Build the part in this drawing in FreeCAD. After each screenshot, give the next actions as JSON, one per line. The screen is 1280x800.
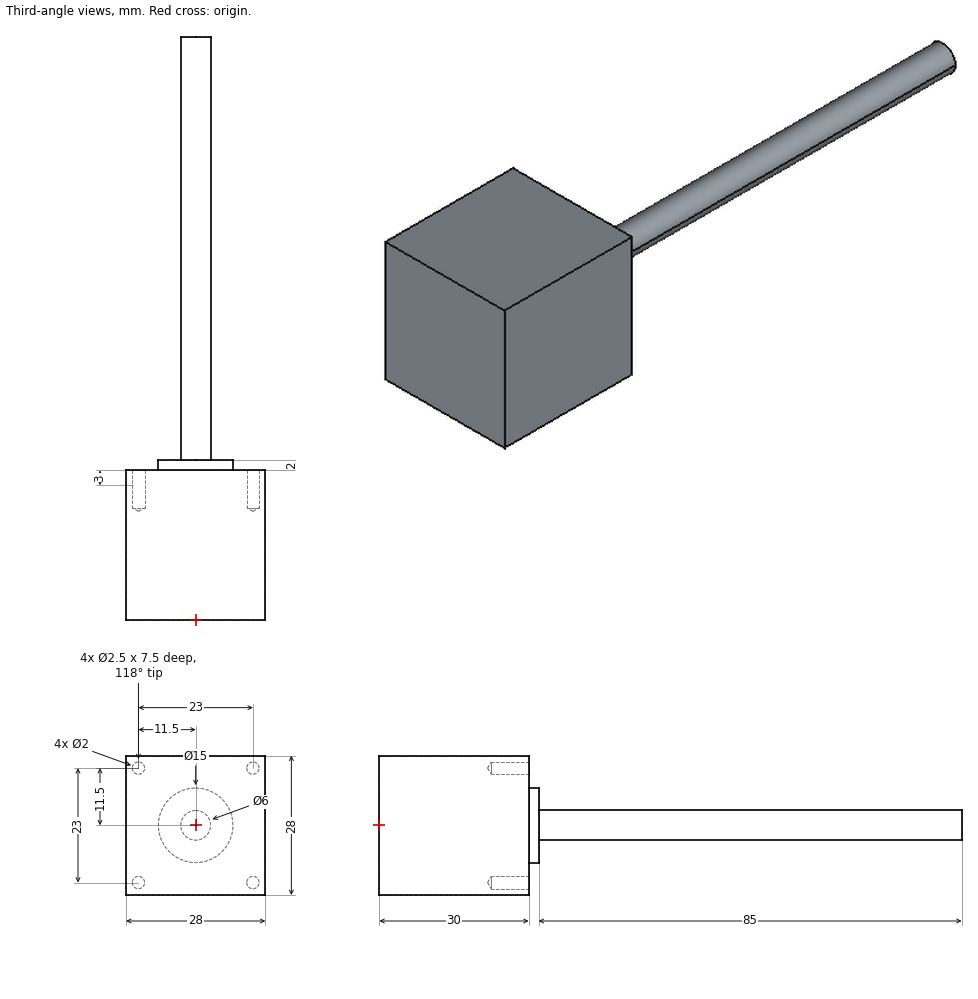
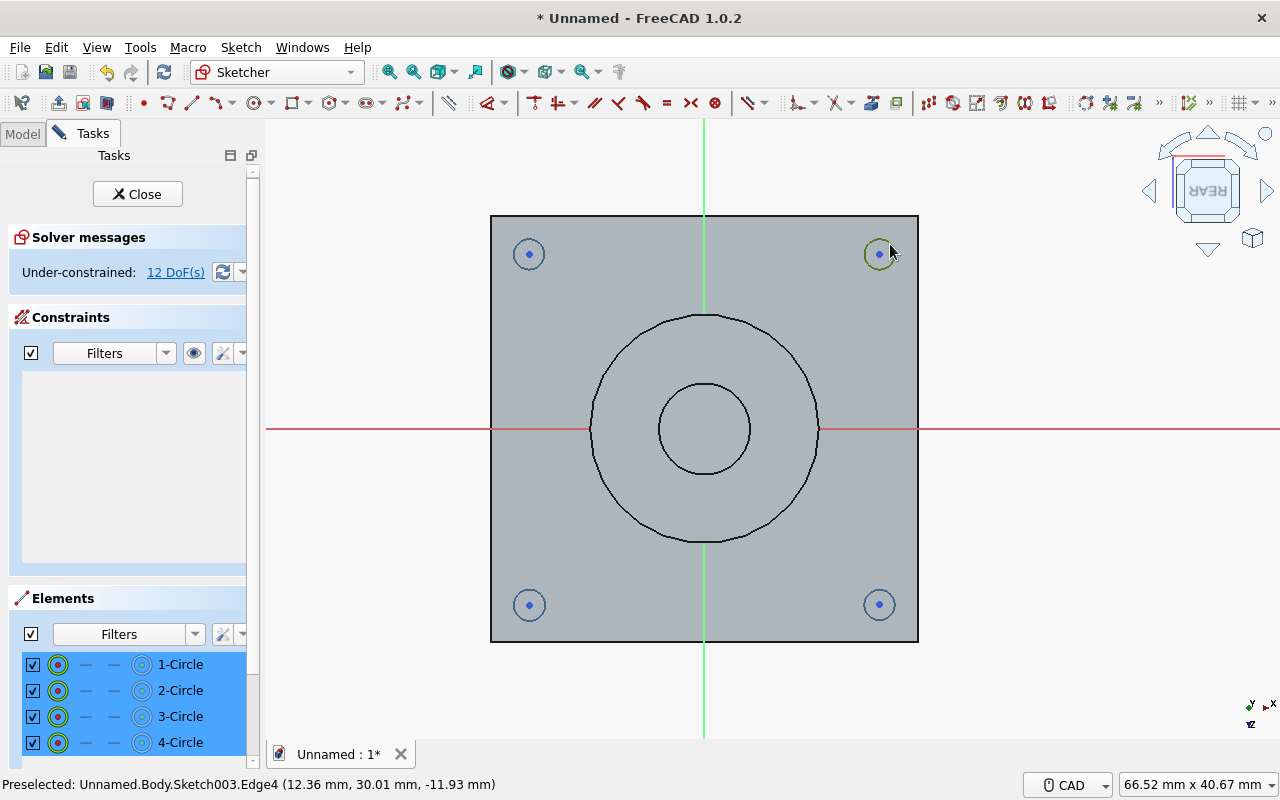
{"action": "left_click", "coordinate": [668, 104]}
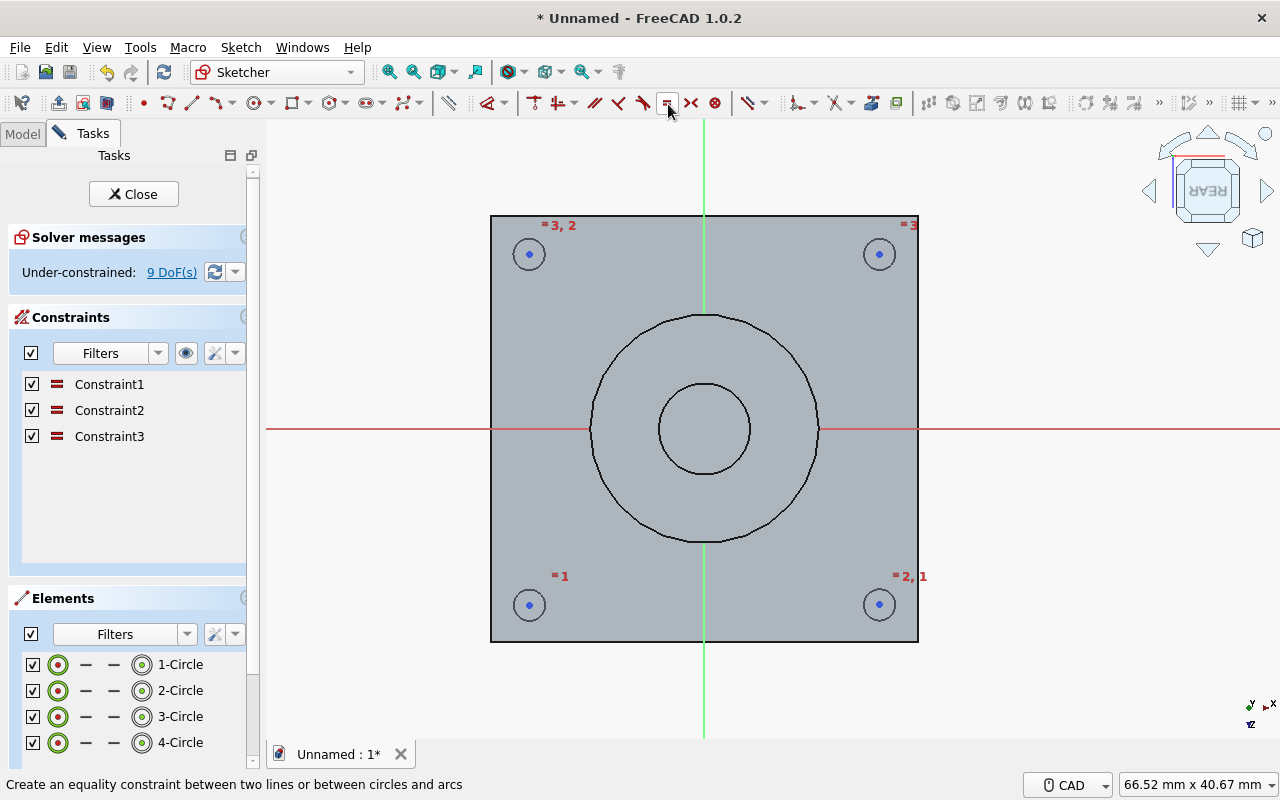
{"action": "left_click", "coordinate": [529, 605]}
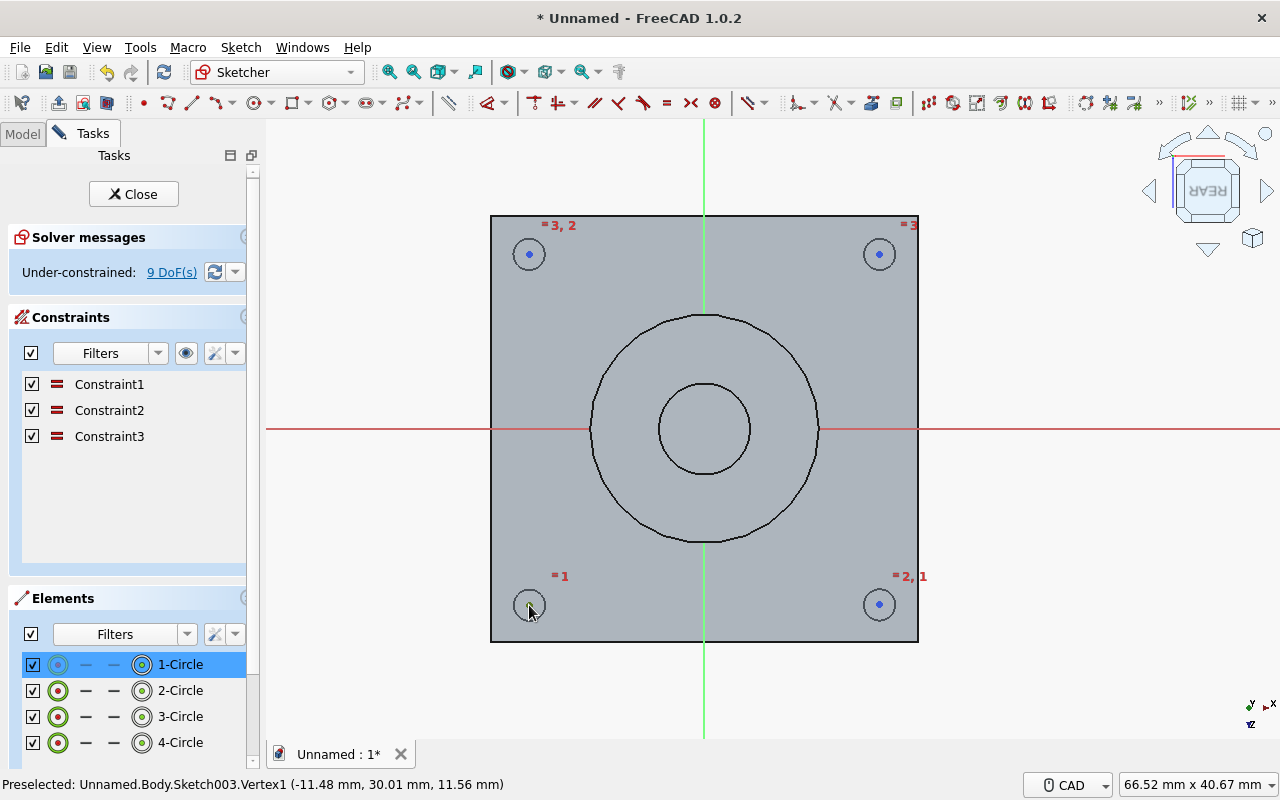
{"action": "left_click", "coordinate": [880, 605]}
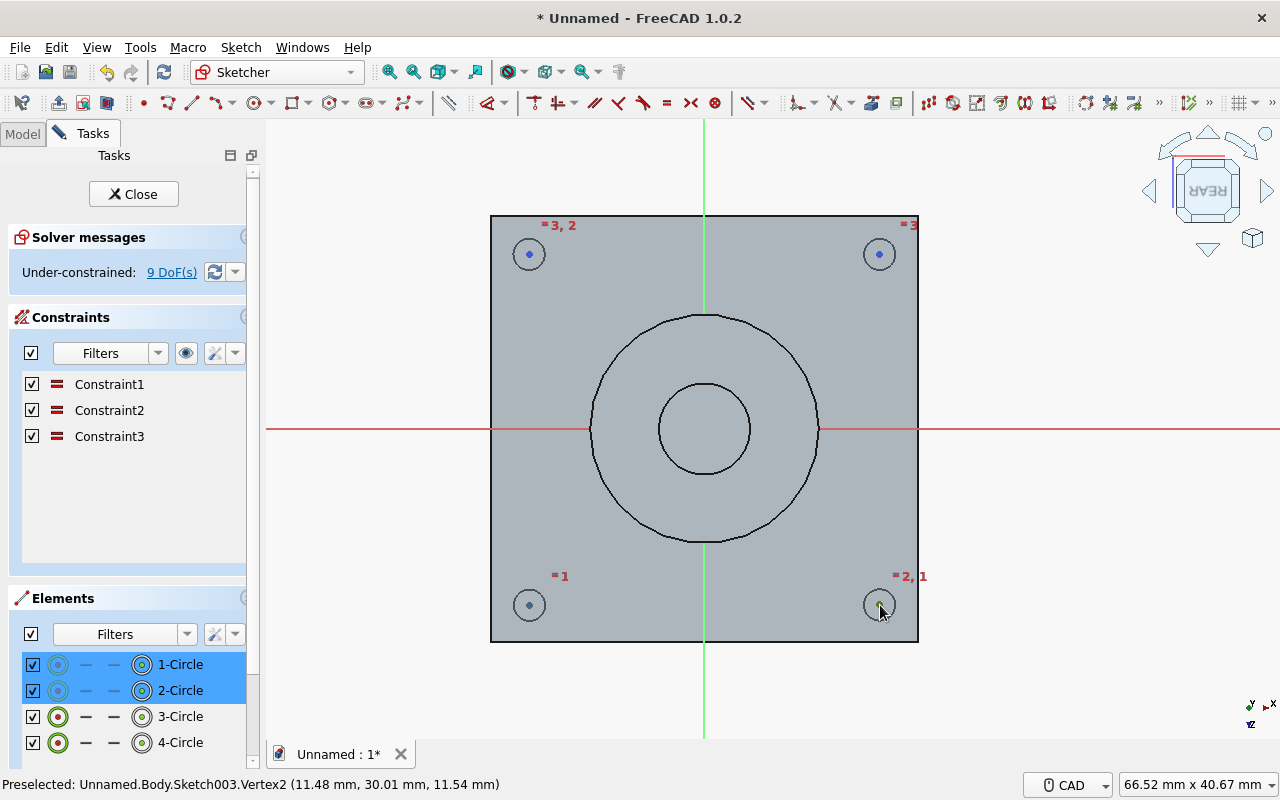
{"action": "left_click", "coordinate": [576, 104]}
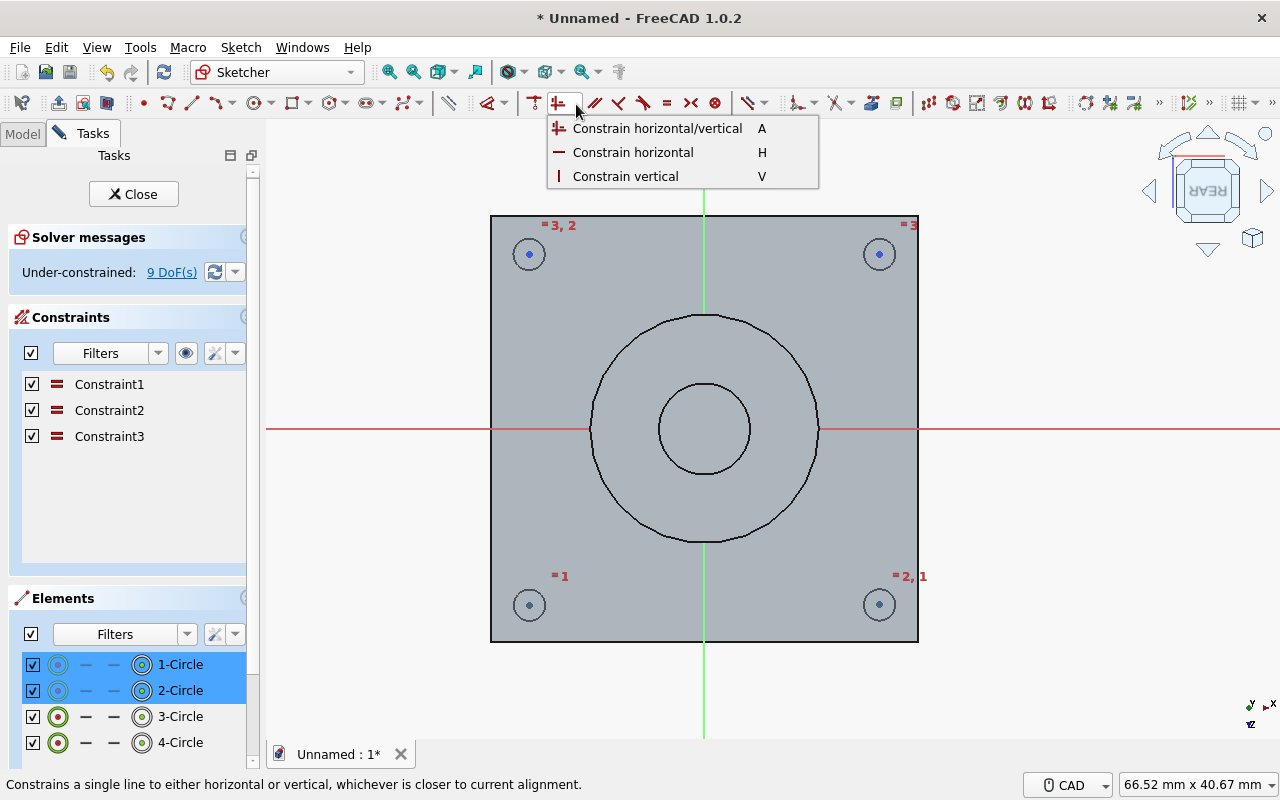
{"action": "left_click", "coordinate": [683, 152]}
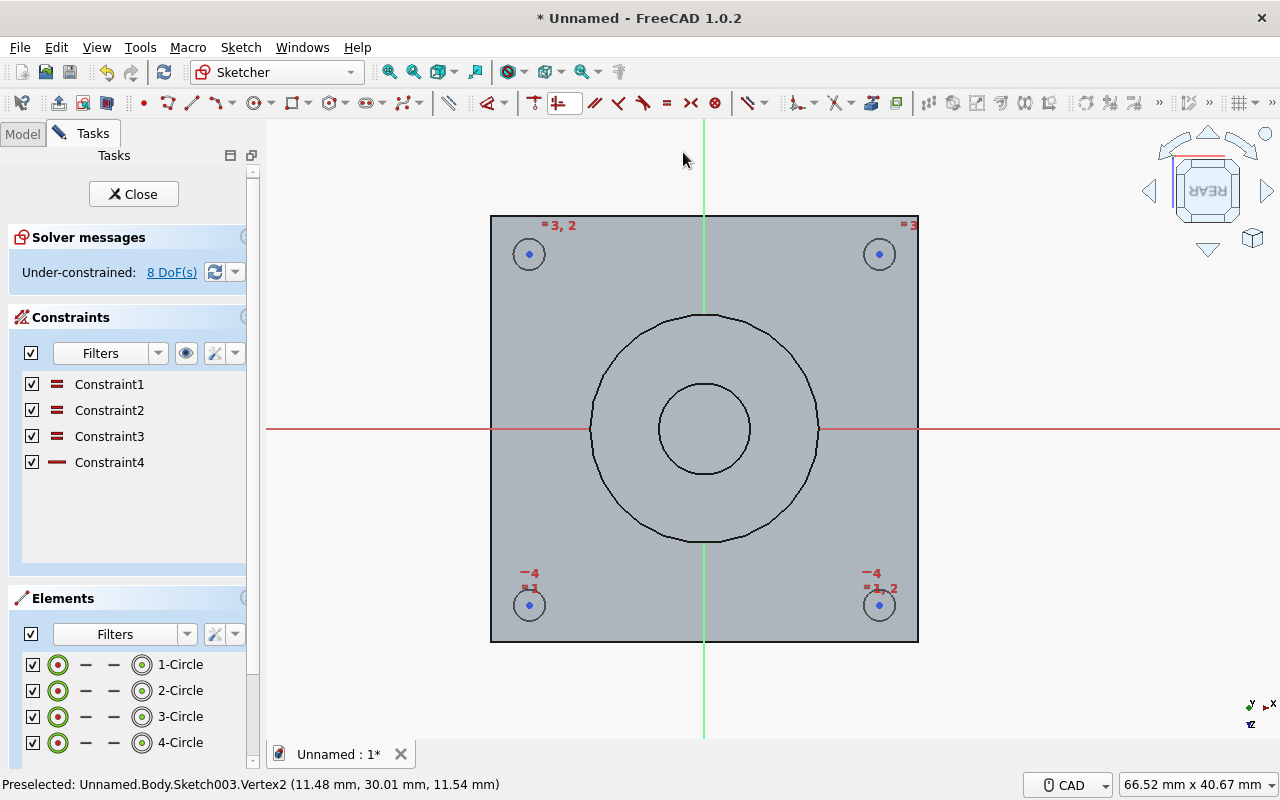
{"action": "left_click", "coordinate": [529, 605]}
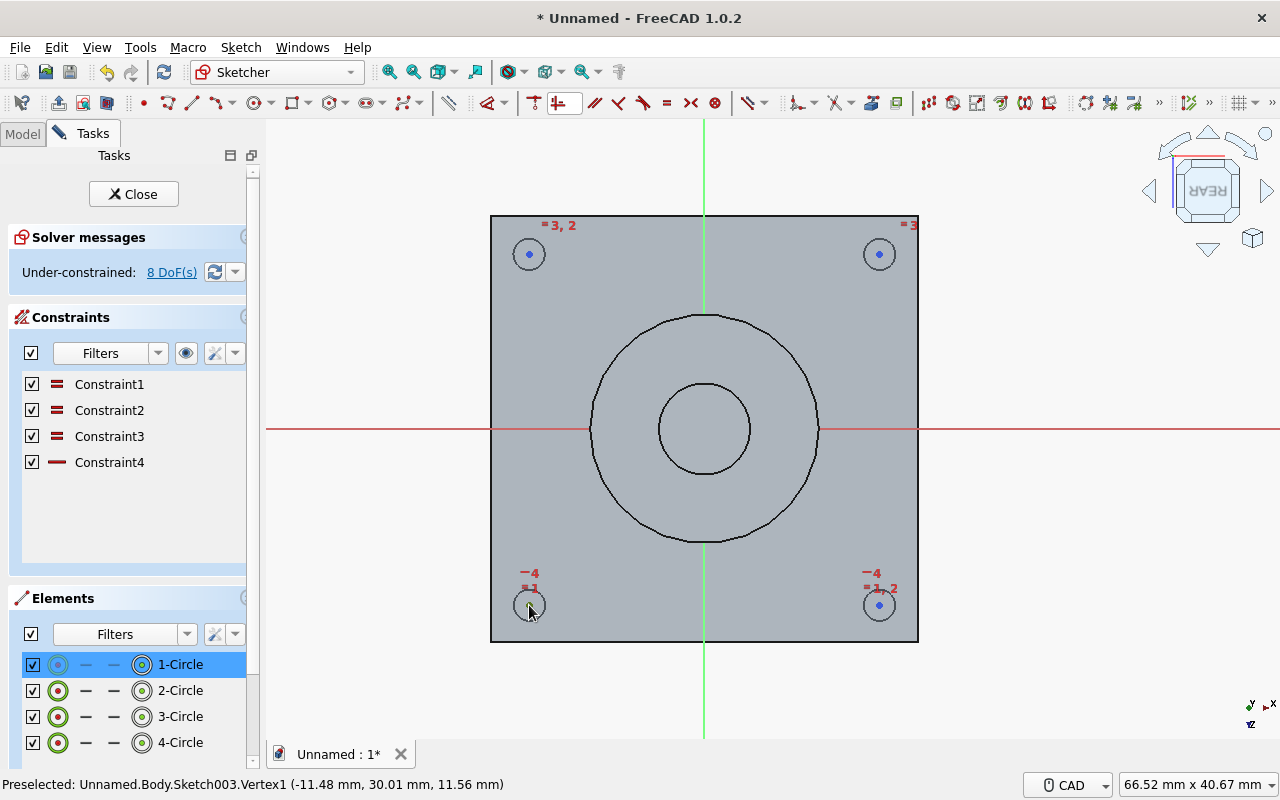
{"action": "left_click", "coordinate": [529, 254]}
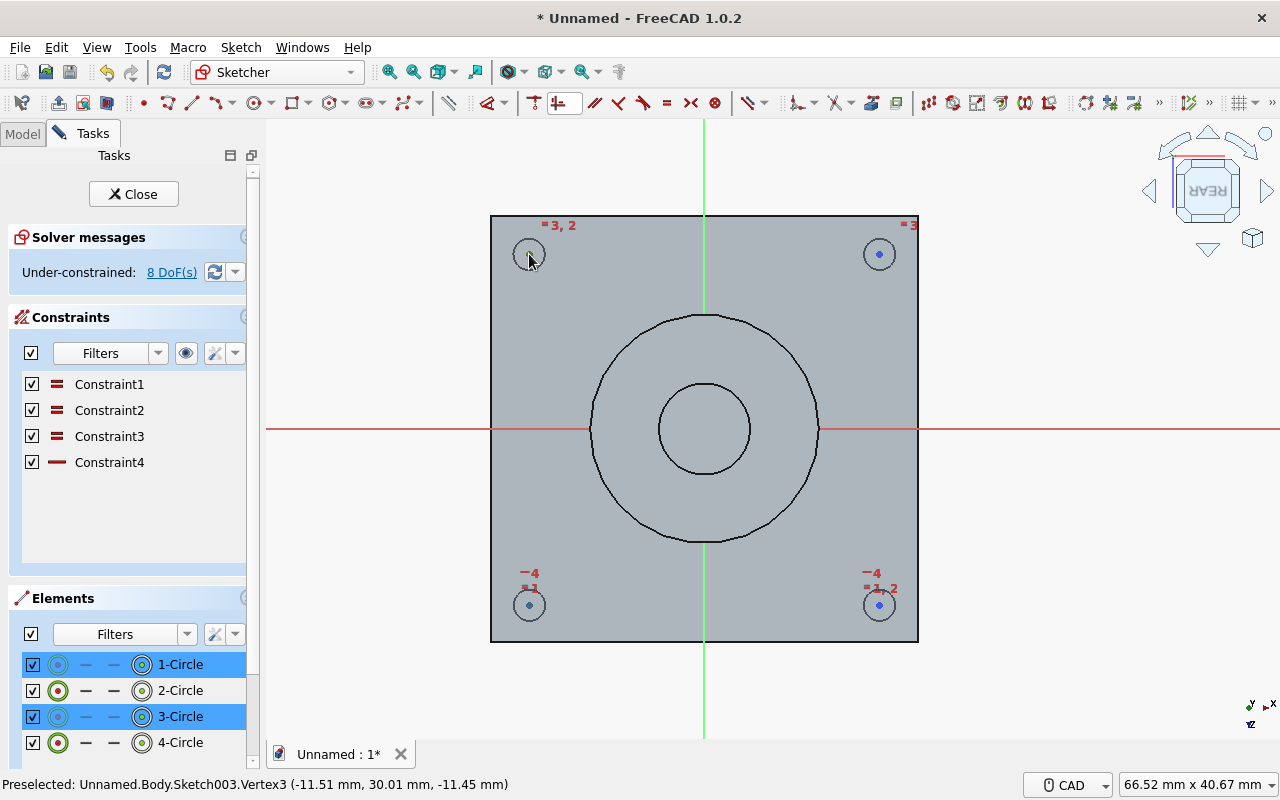
{"action": "key", "text": "v"}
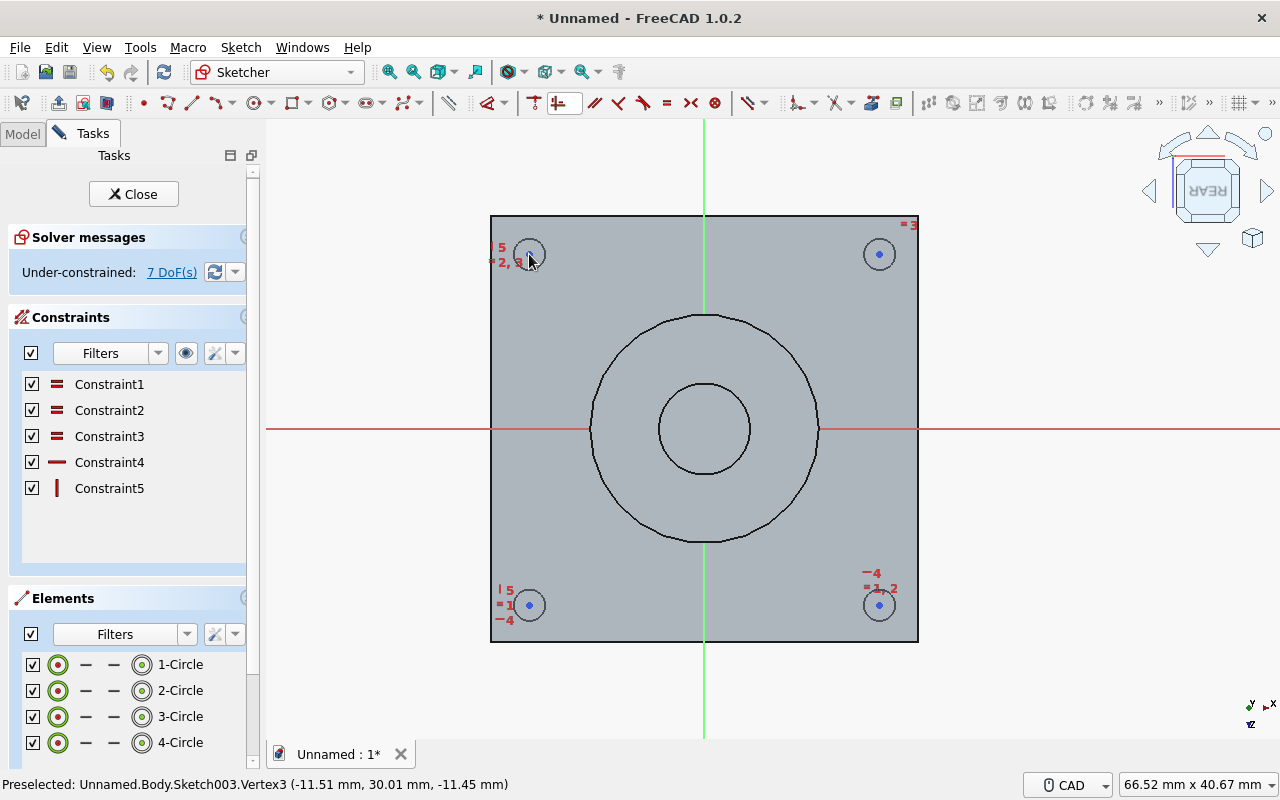
{"action": "left_click", "coordinate": [880, 605]}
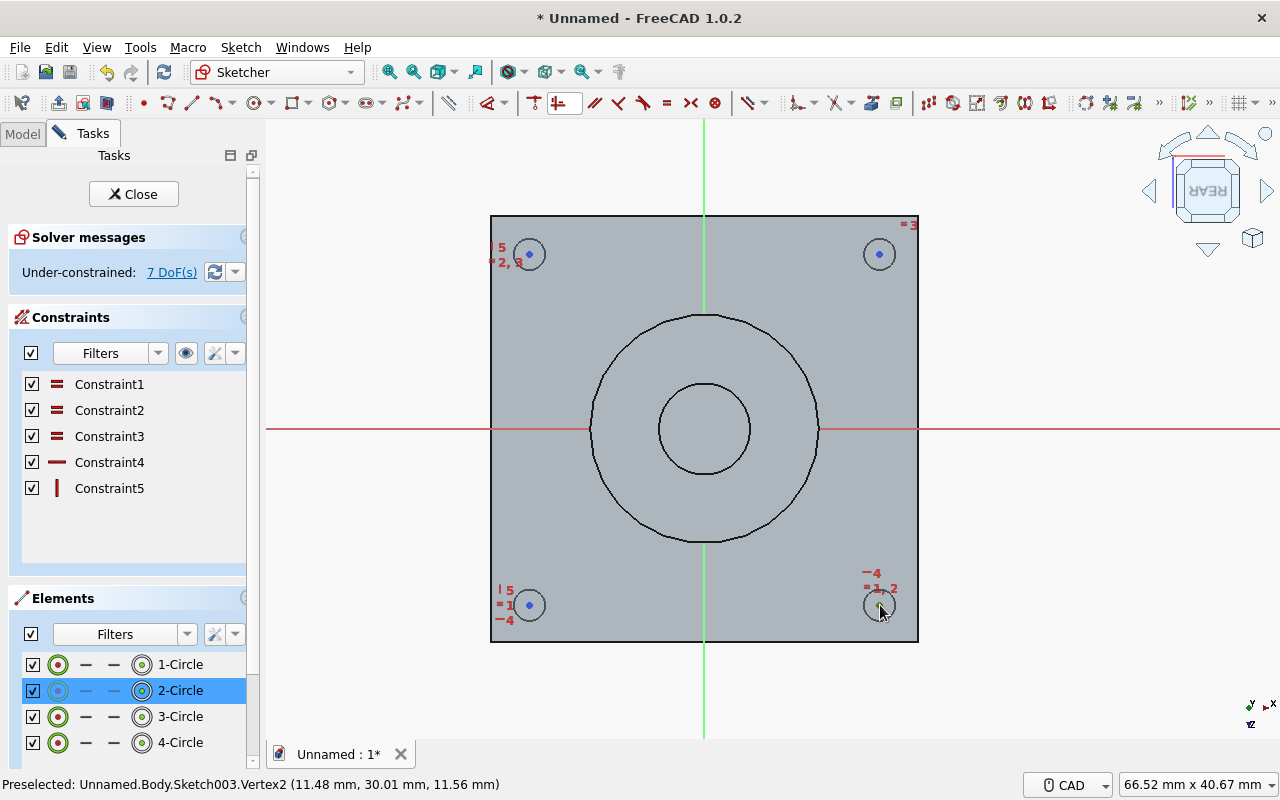
{"action": "left_click", "coordinate": [880, 254]}